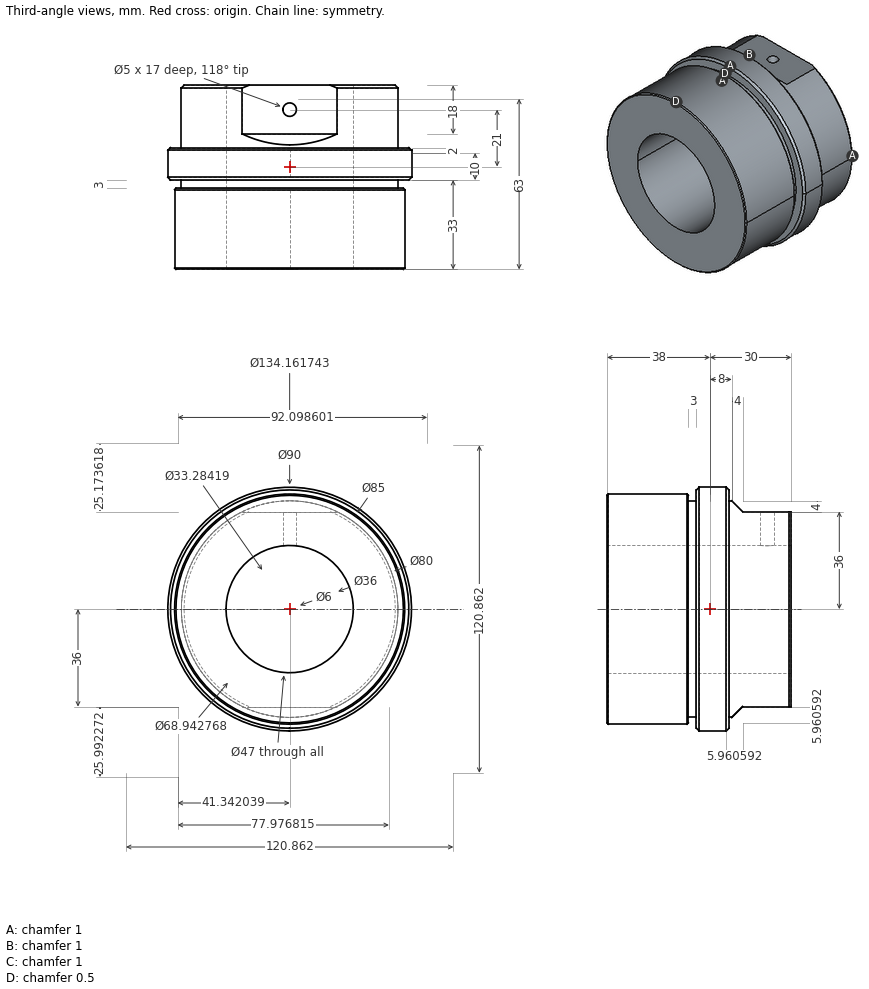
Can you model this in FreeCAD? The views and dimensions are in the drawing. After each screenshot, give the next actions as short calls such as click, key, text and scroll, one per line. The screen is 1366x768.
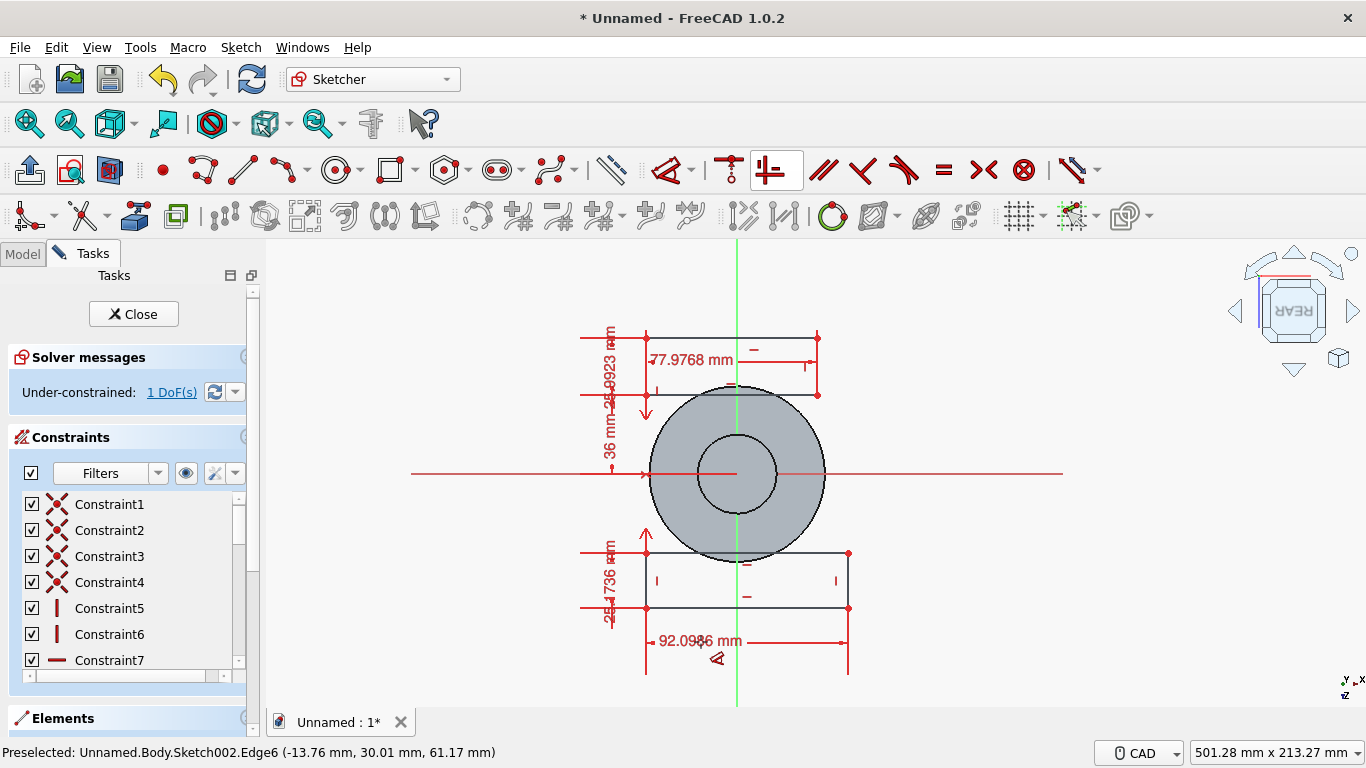
click(646, 338)
click(692, 304)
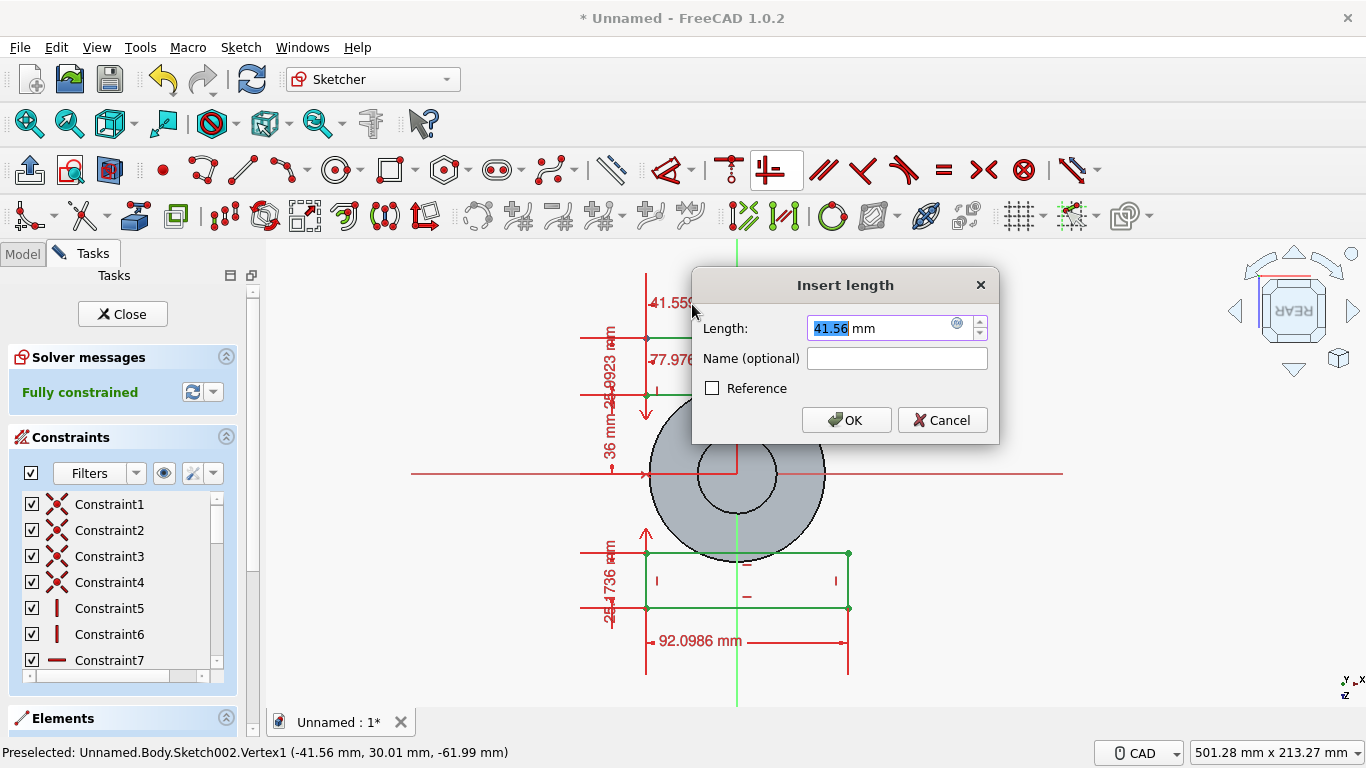
text(41.342039)
key(Return)
key(Escape)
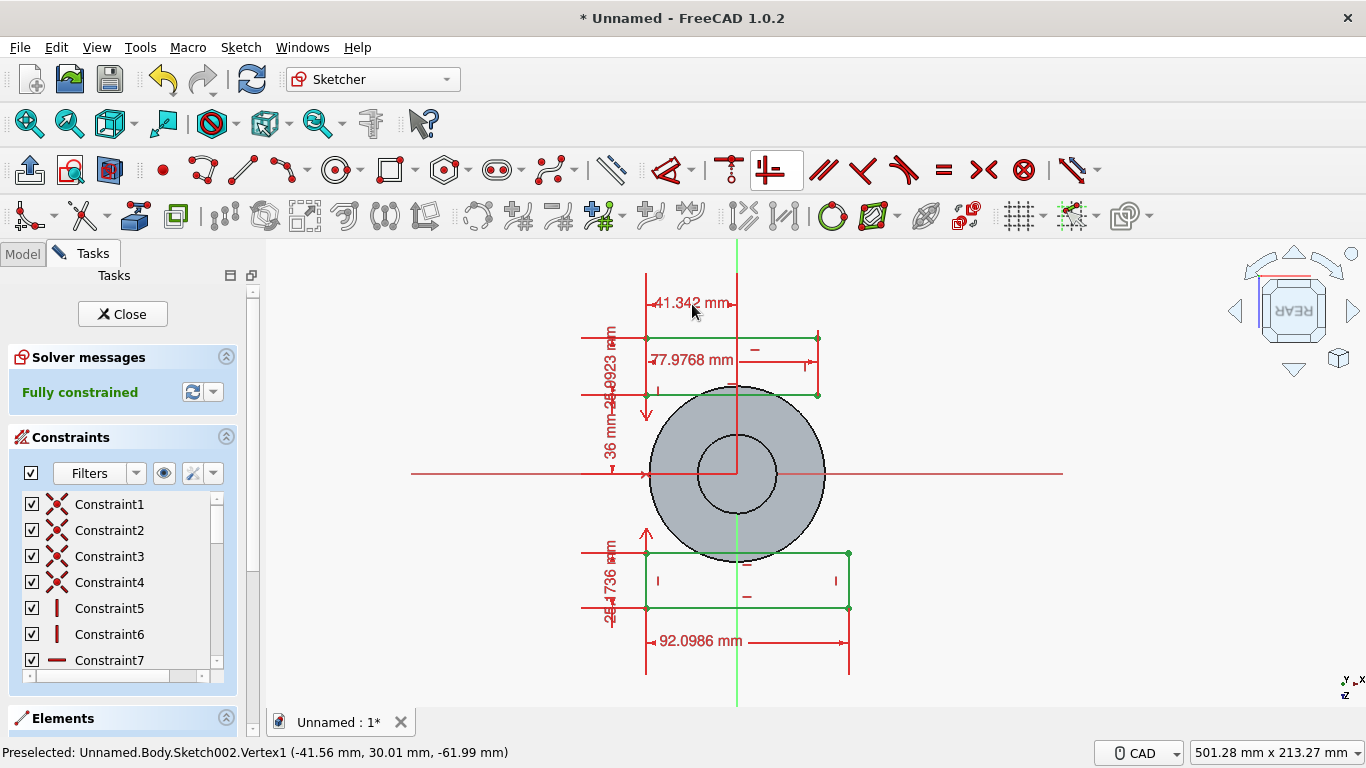
click(123, 314)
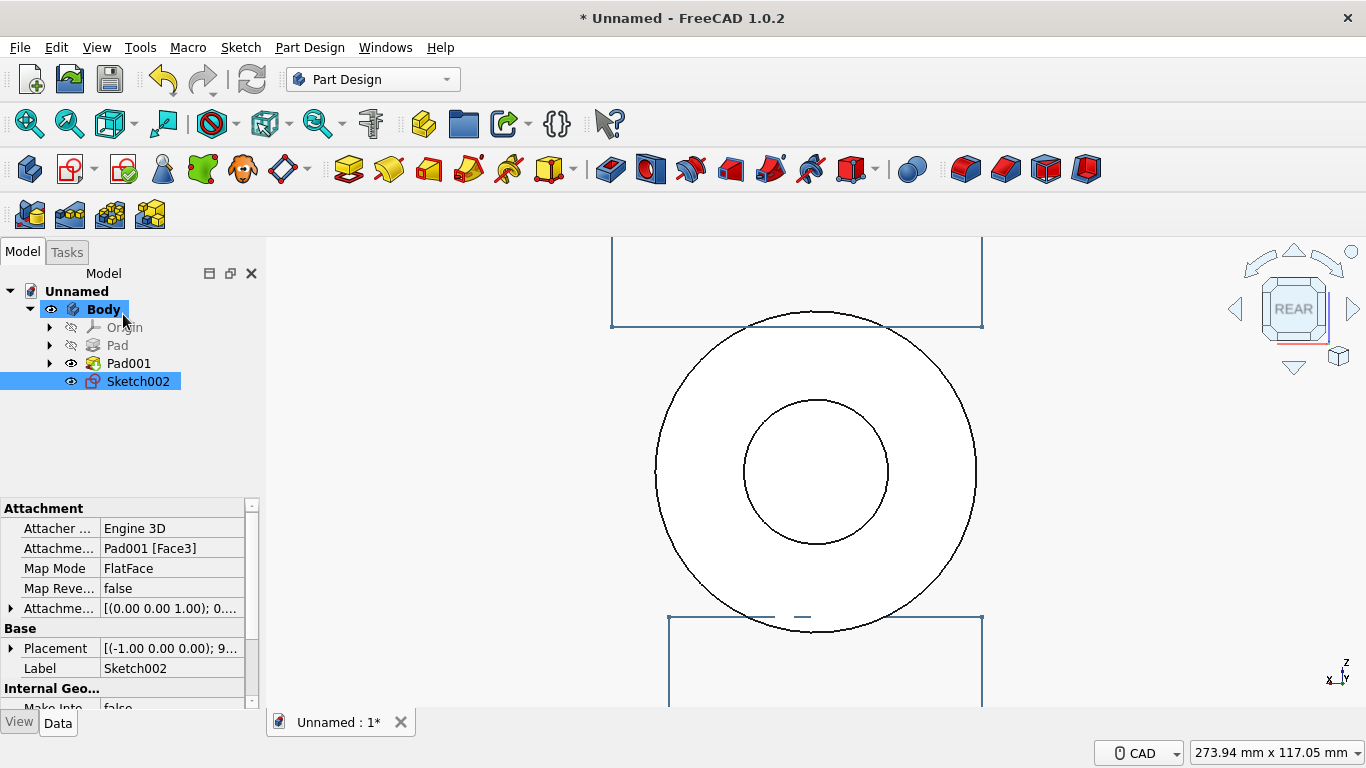
click(612, 170)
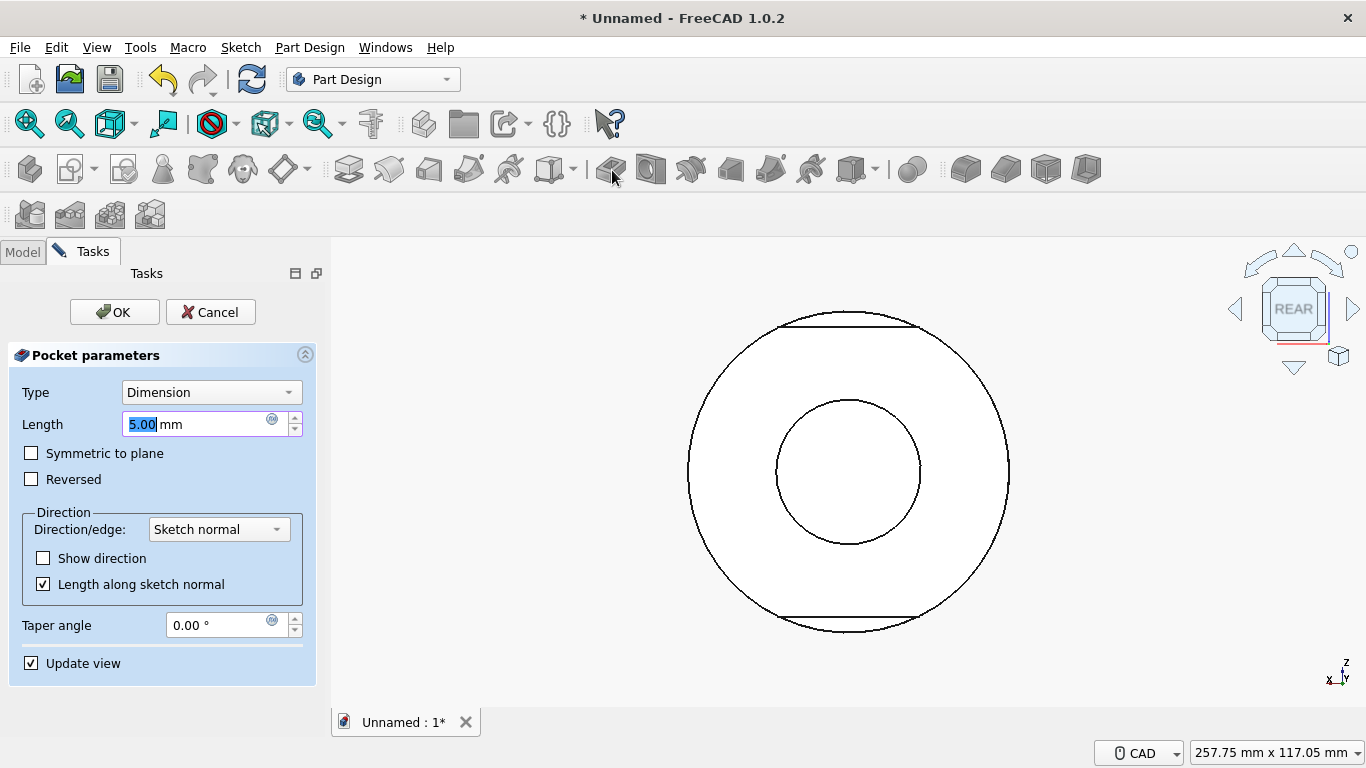
text(18)
key(Tab)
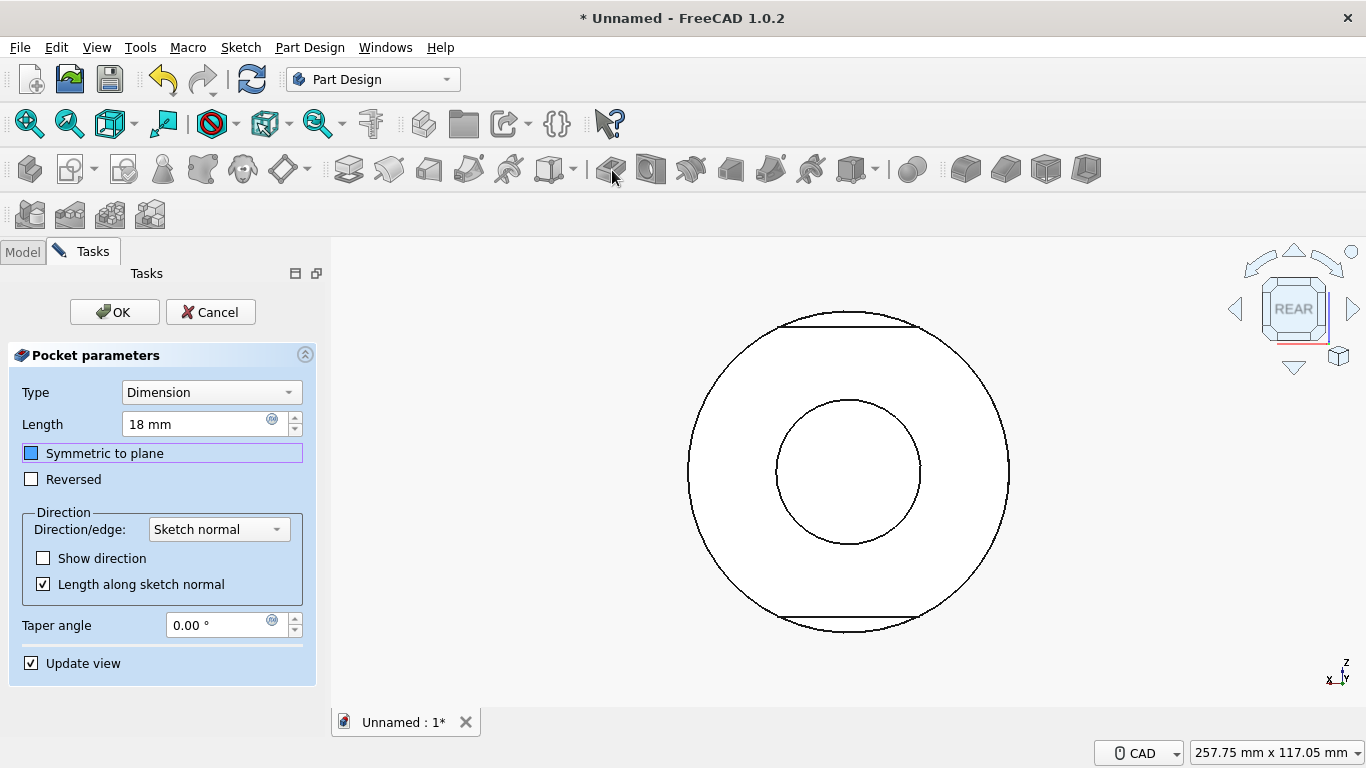
click(115, 312)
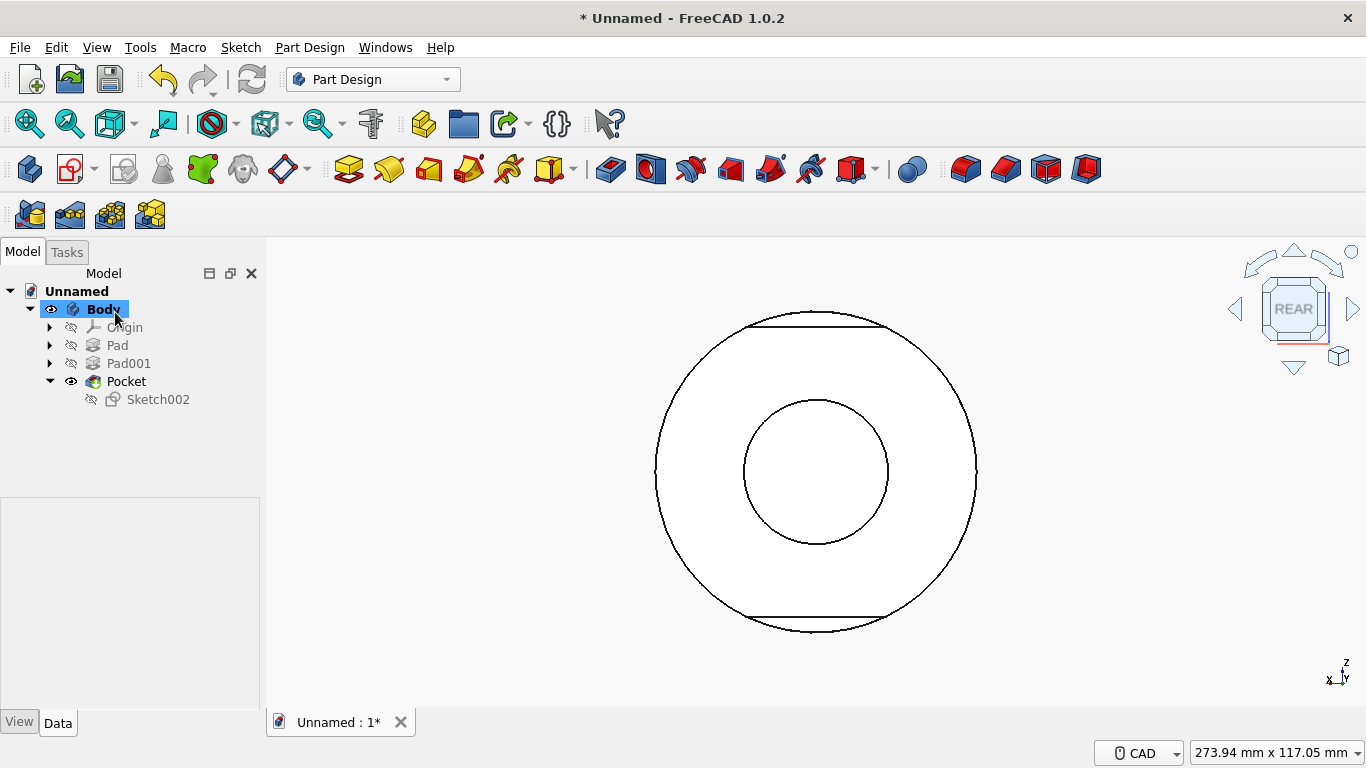
click(70, 170)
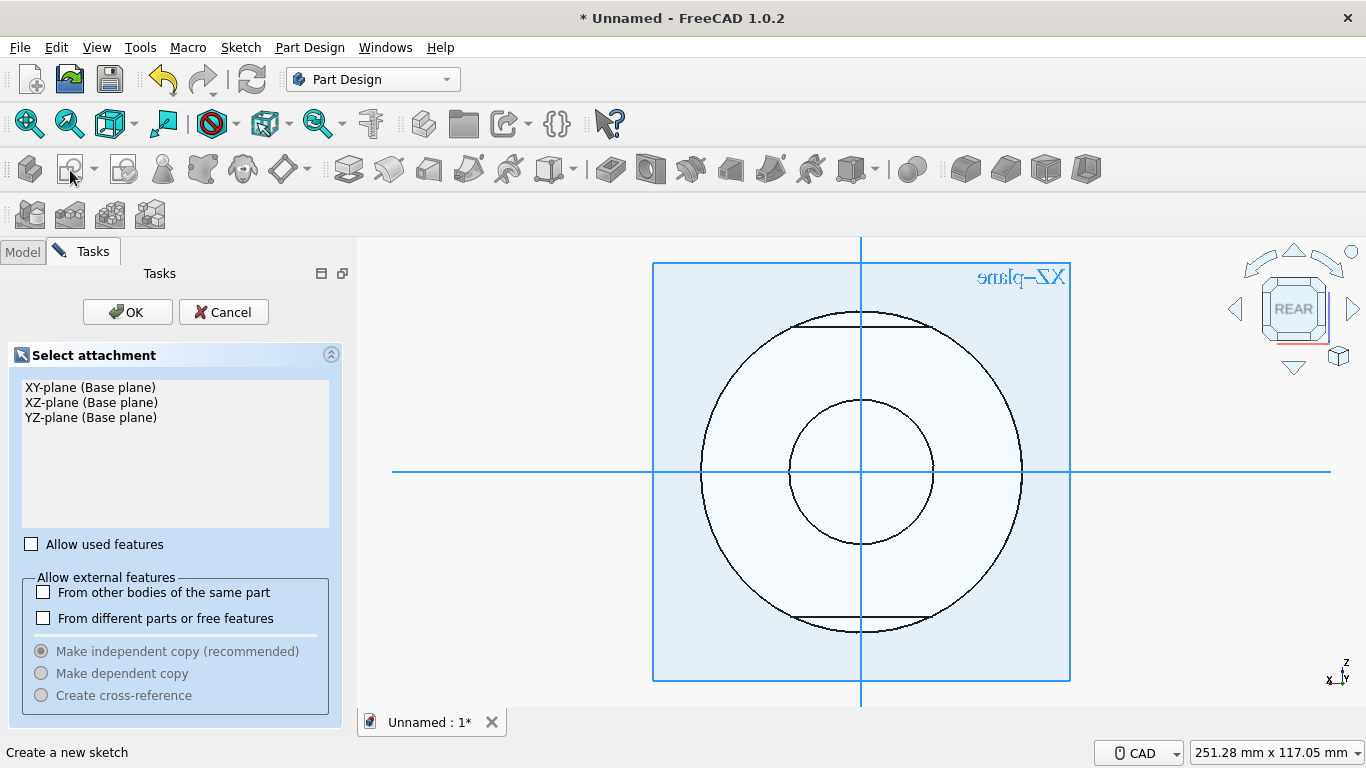
click(82, 402)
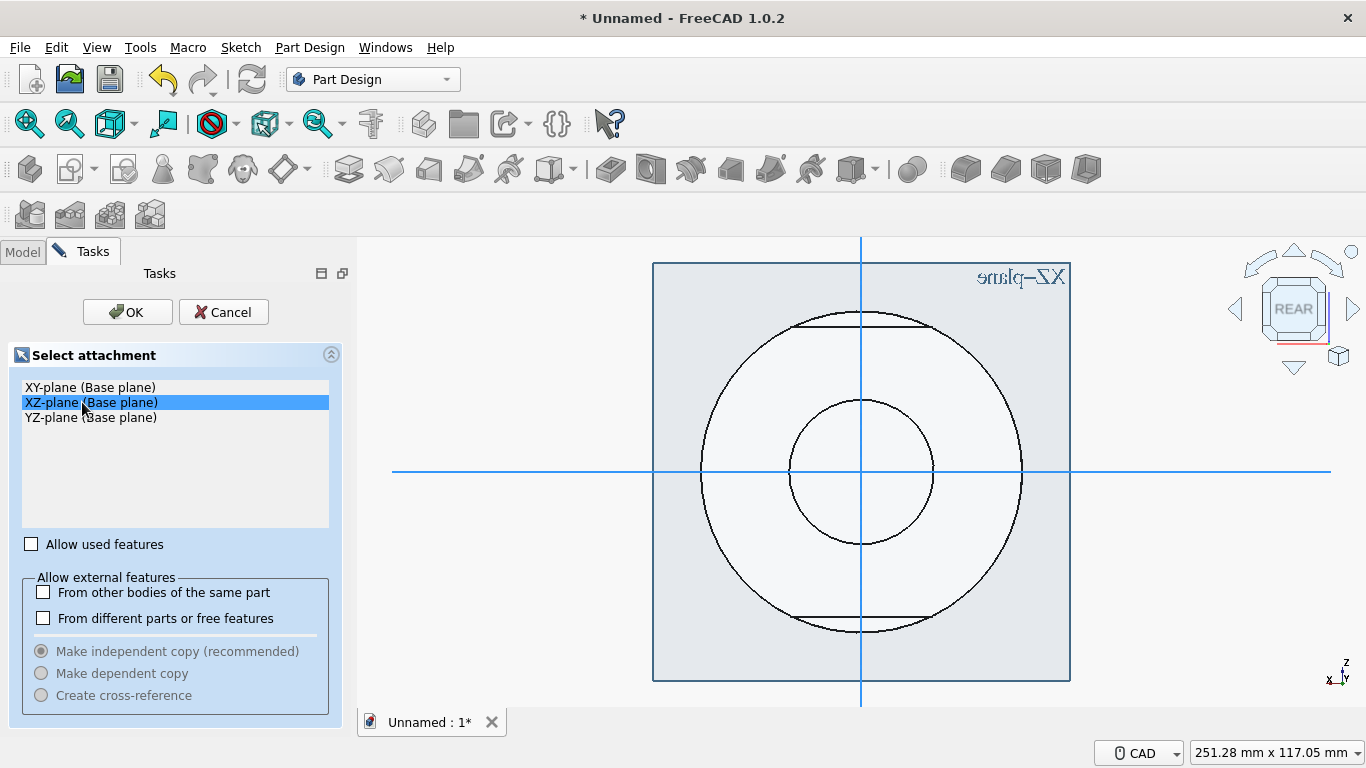
click(128, 312)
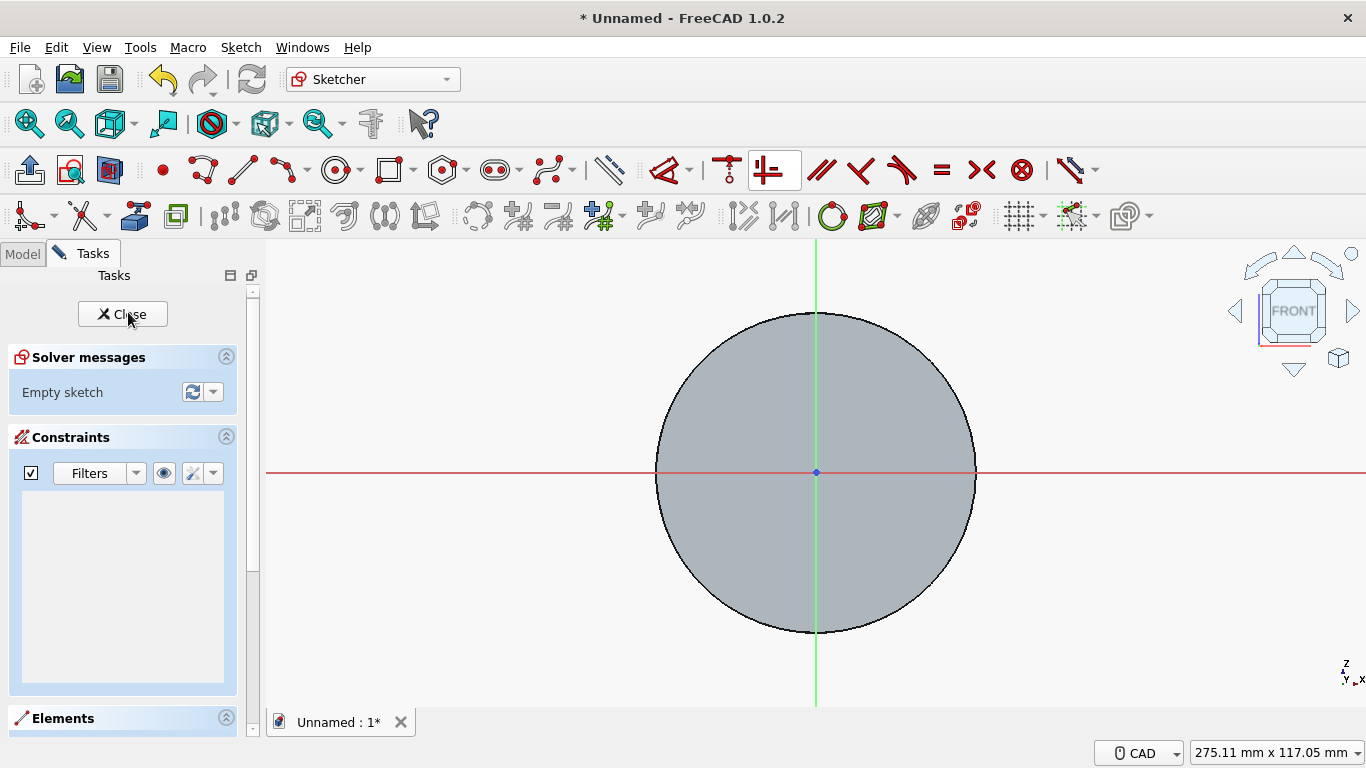
click(336, 170)